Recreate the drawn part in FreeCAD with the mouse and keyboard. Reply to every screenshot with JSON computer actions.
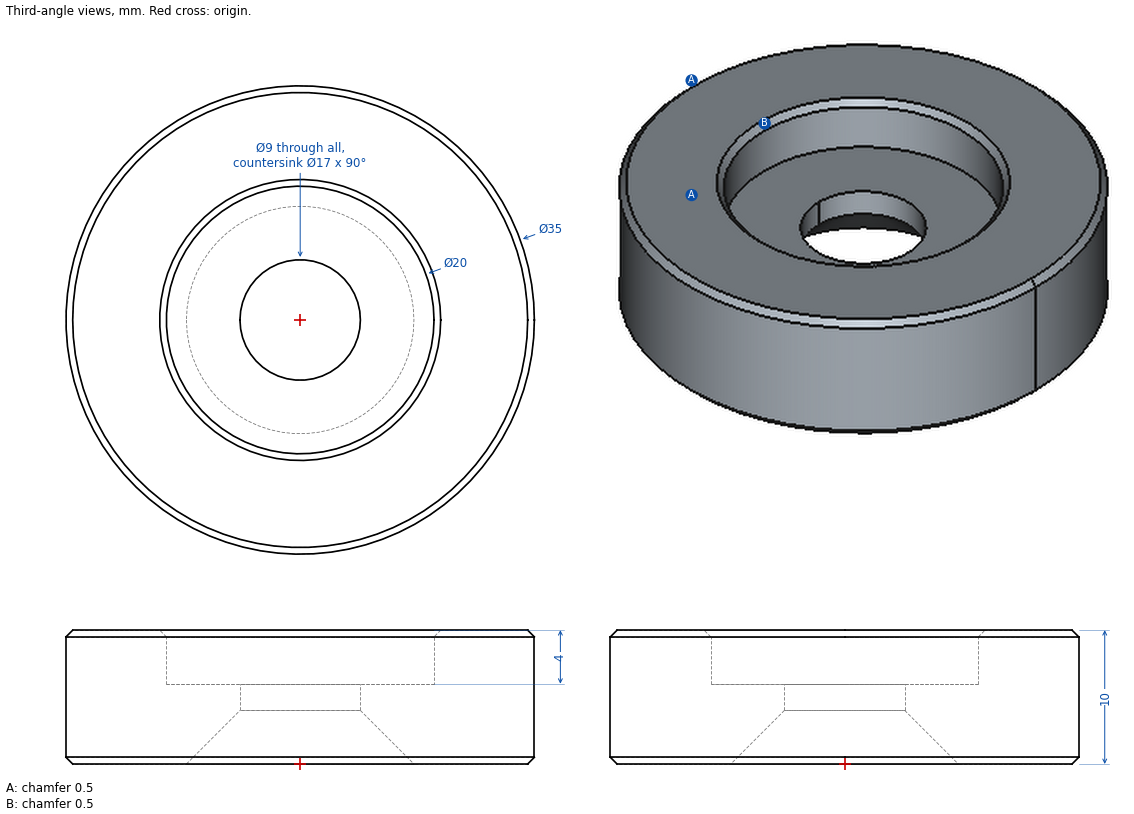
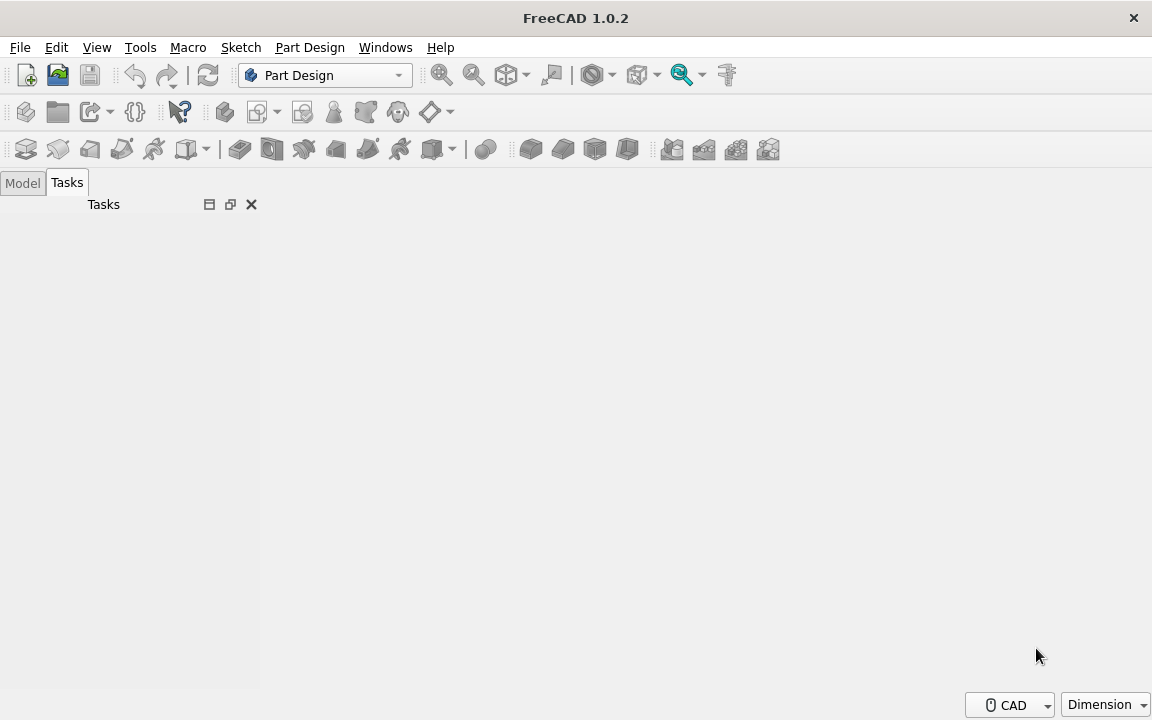
{"action": "left_click", "coordinate": [26, 76]}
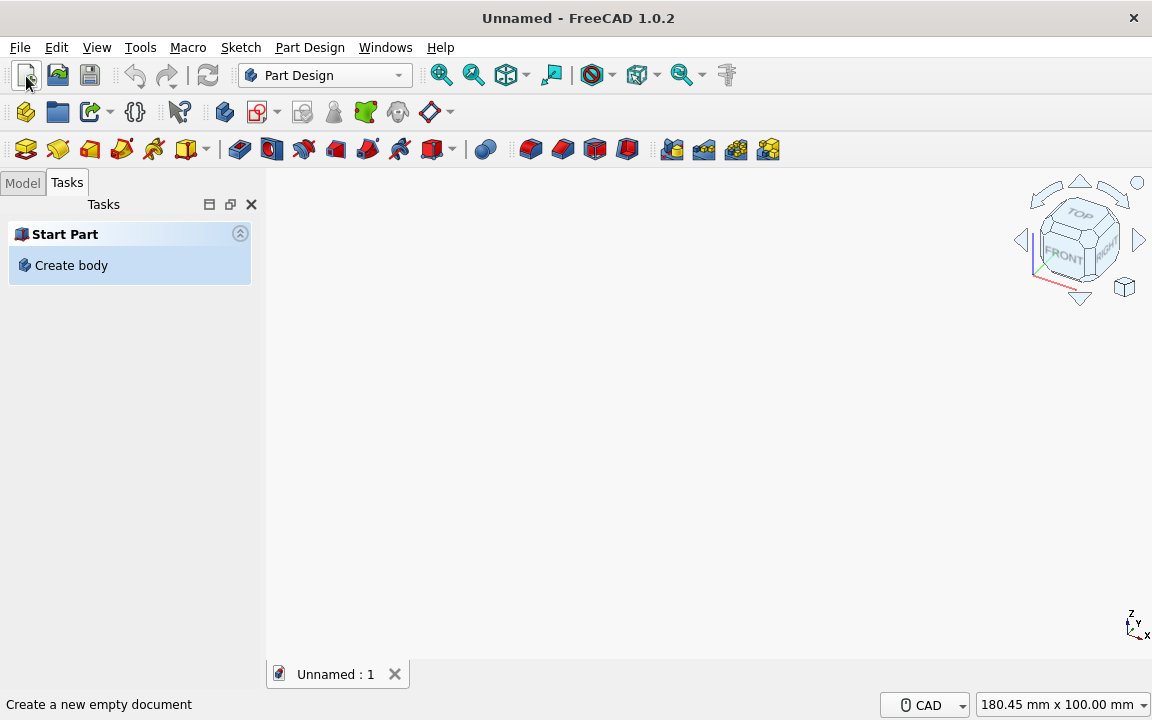
{"action": "left_click", "coordinate": [258, 112]}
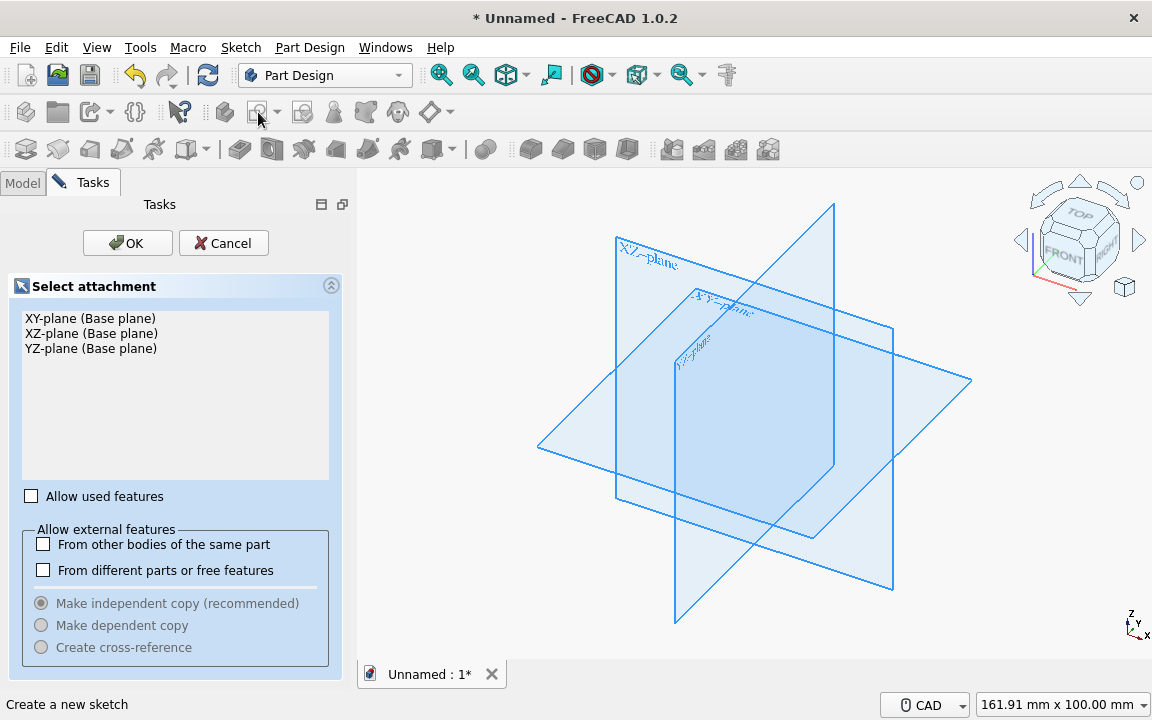
{"action": "left_click", "coordinate": [82, 318]}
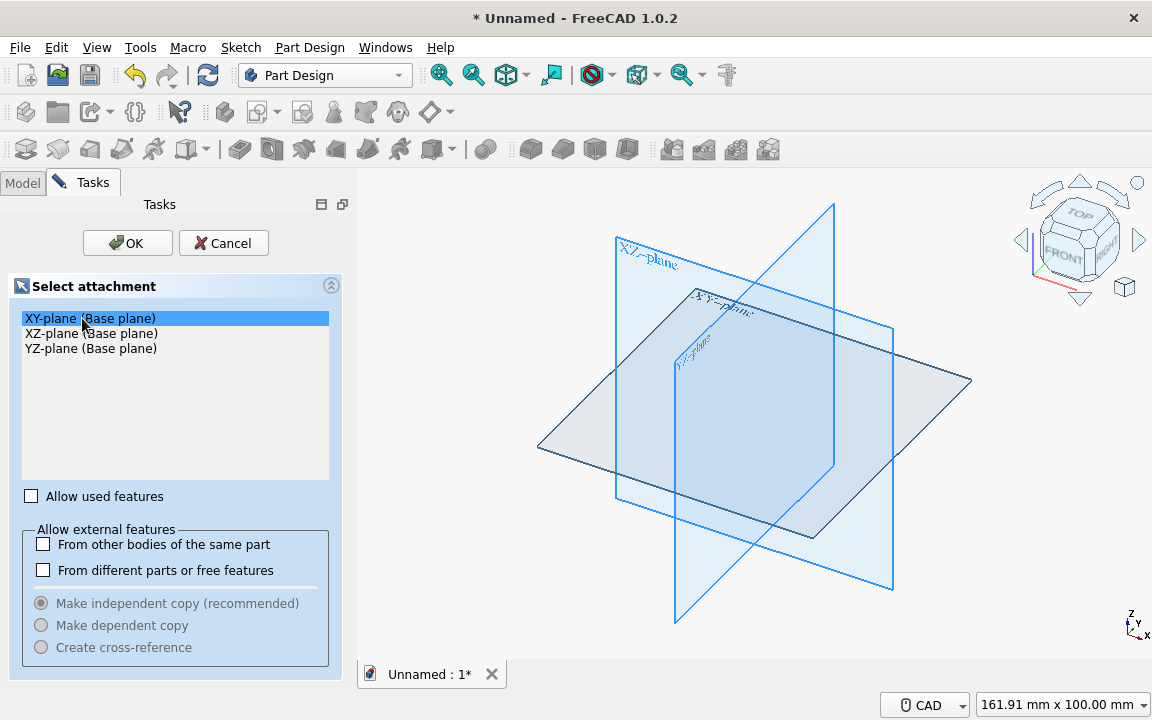
{"action": "left_click", "coordinate": [128, 243]}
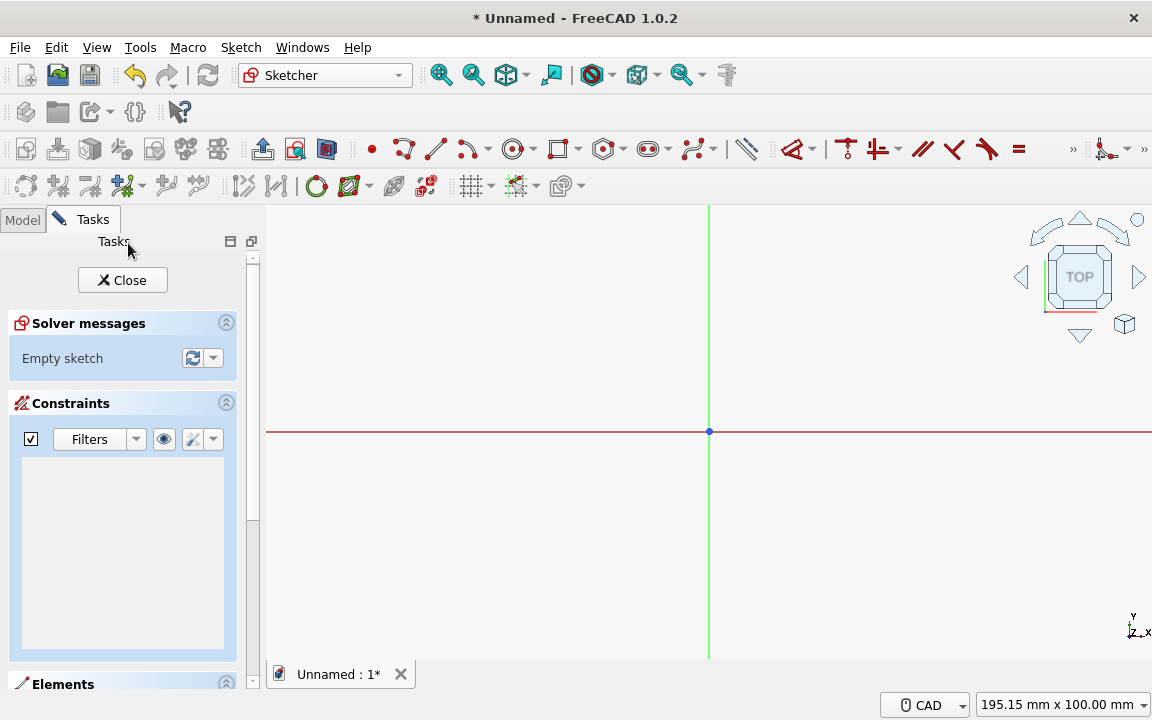
{"action": "scroll", "coordinate": [792, 432], "scroll_direction": "up", "scroll_amount": 3}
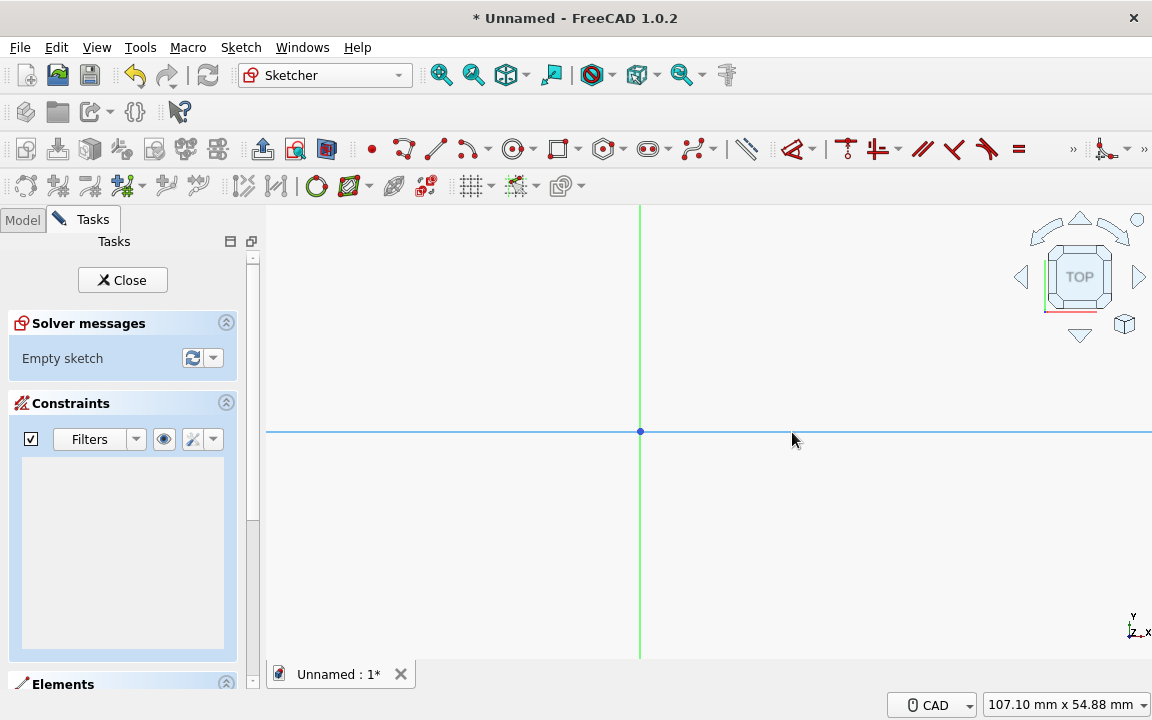
{"action": "left_click", "coordinate": [514, 150]}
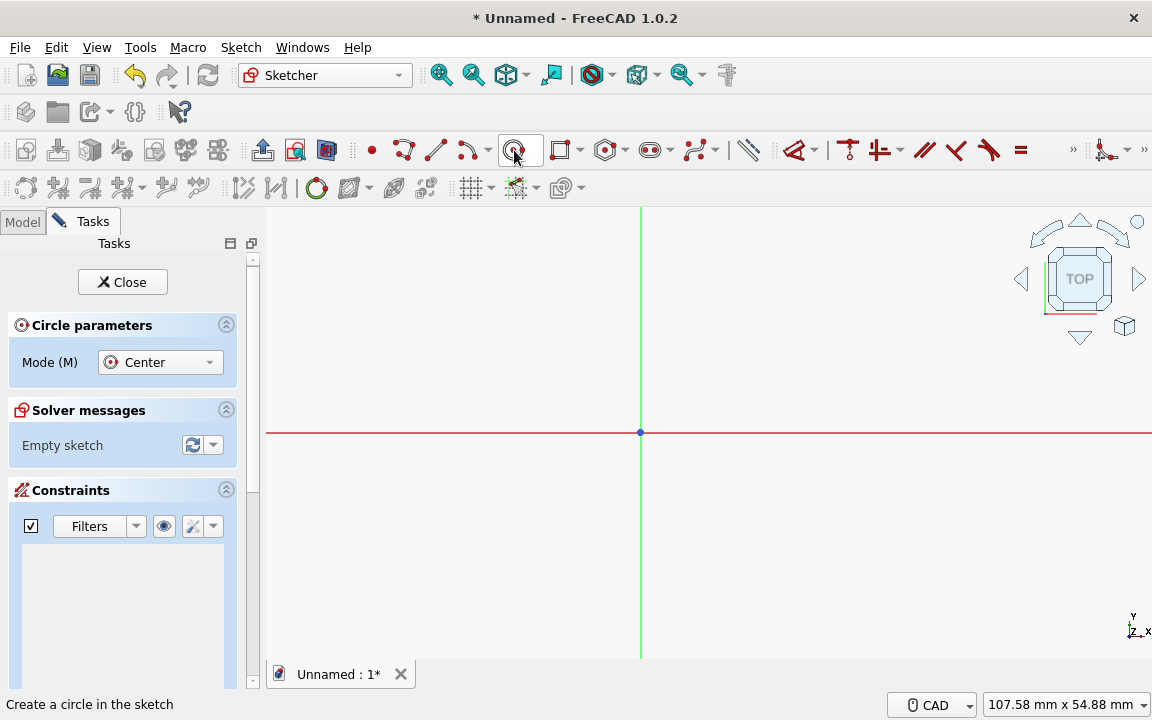
{"action": "left_click", "coordinate": [641, 433]}
{"action": "mouse_move", "coordinate": [742, 331]}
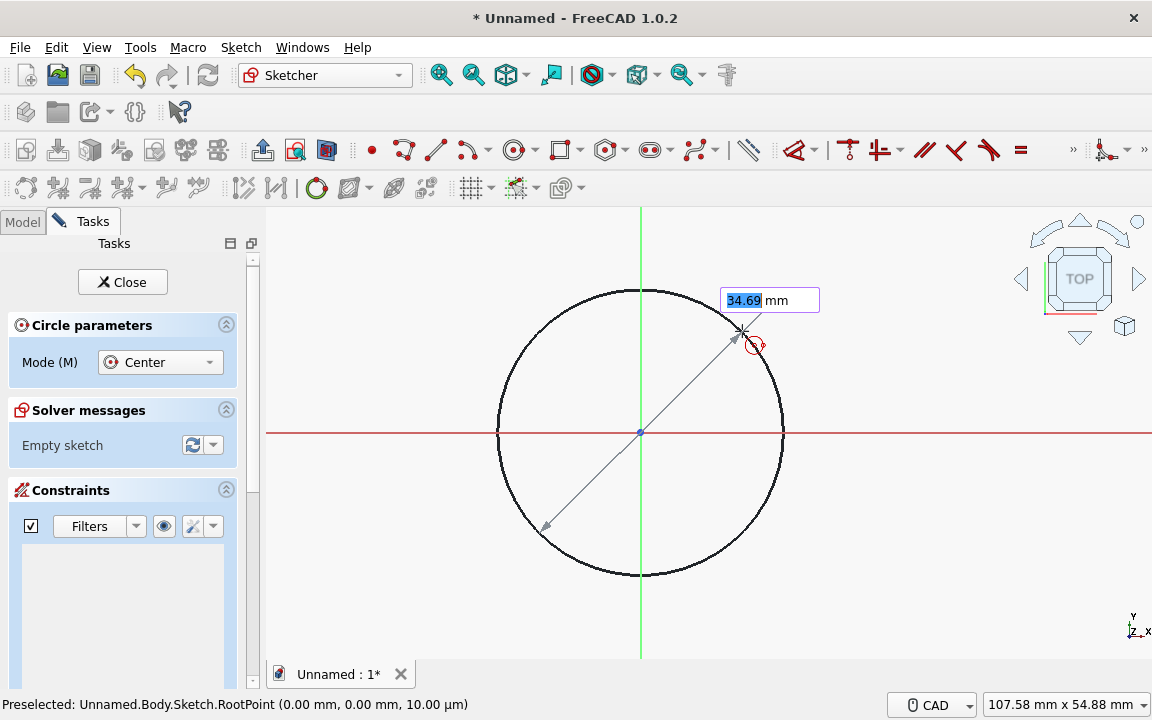
{"action": "type", "text": "35"}
{"action": "key", "text": "Return"}
{"action": "key", "text": "Escape"}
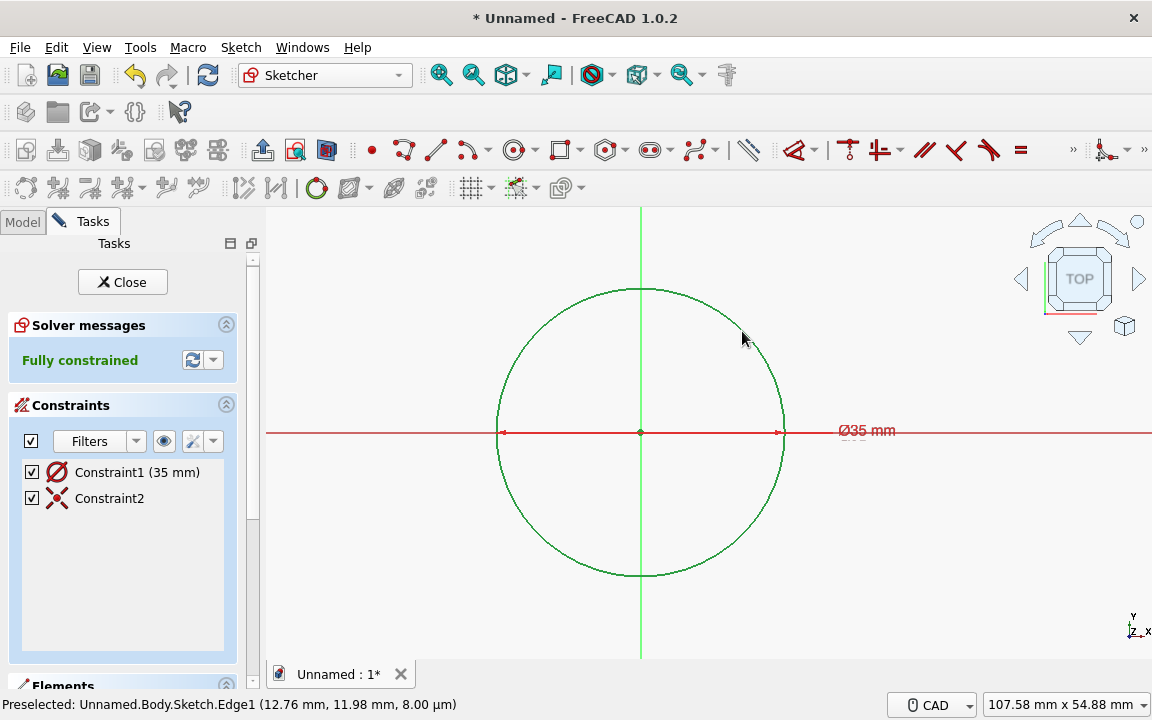
{"action": "left_click", "coordinate": [123, 282]}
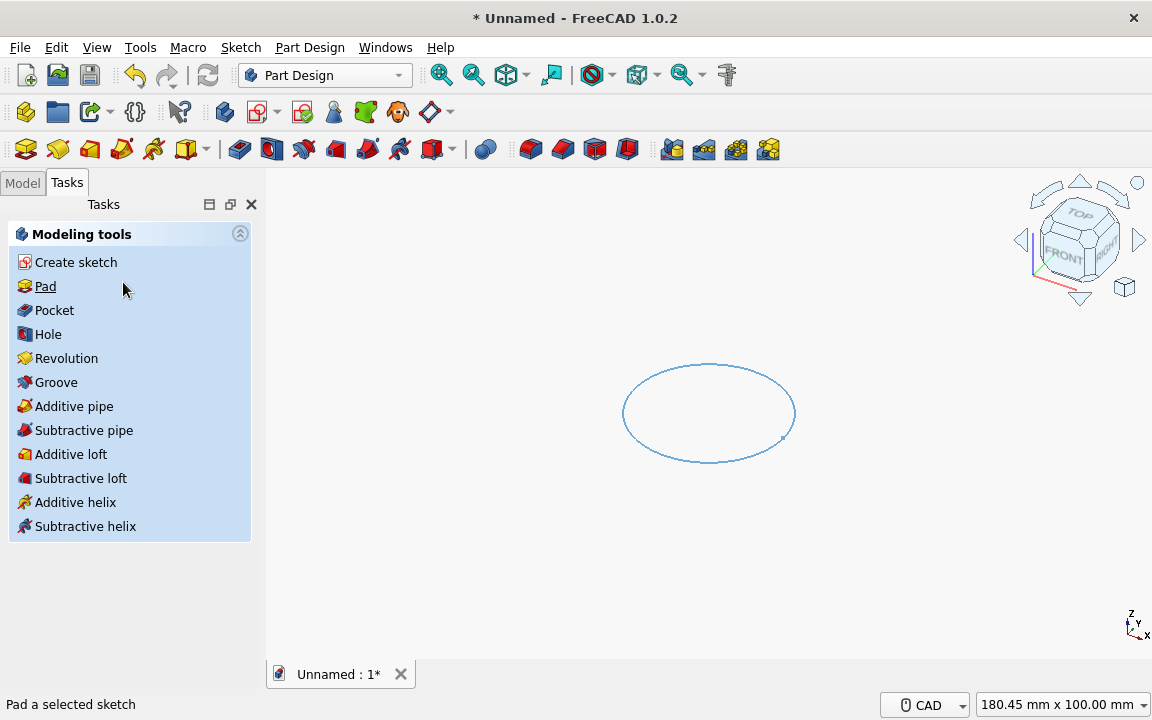
{"action": "left_click", "coordinate": [26, 150]}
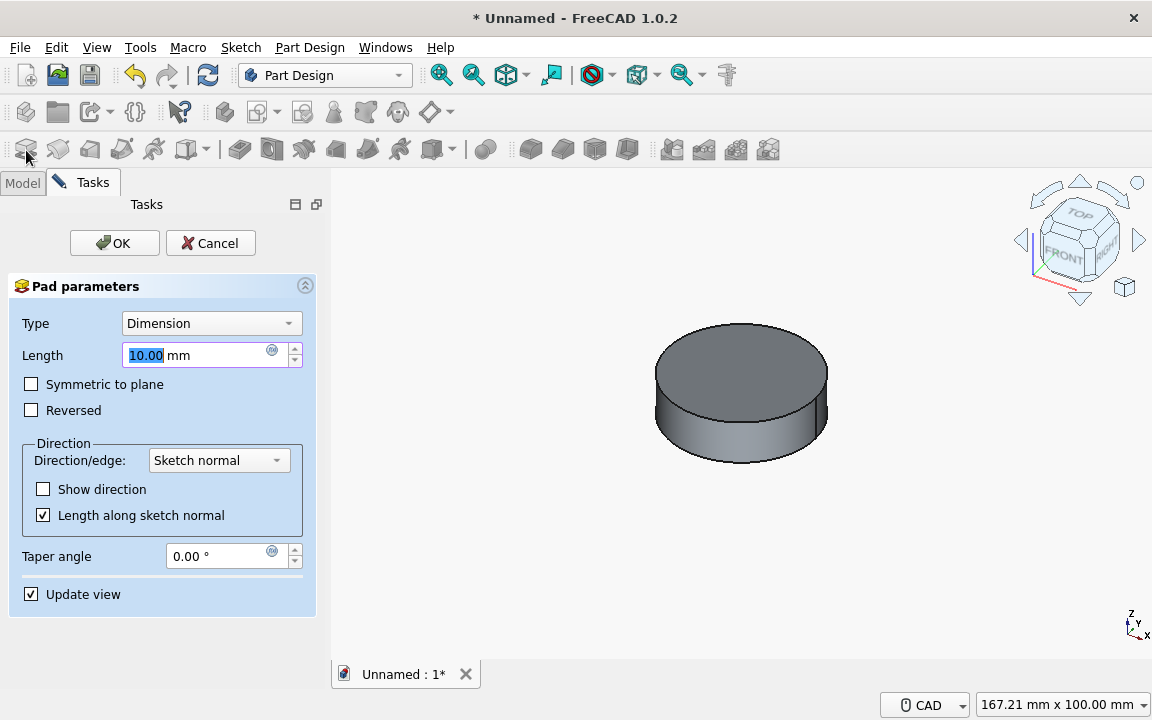
{"action": "type", "text": "10"}
{"action": "key", "text": "Tab"}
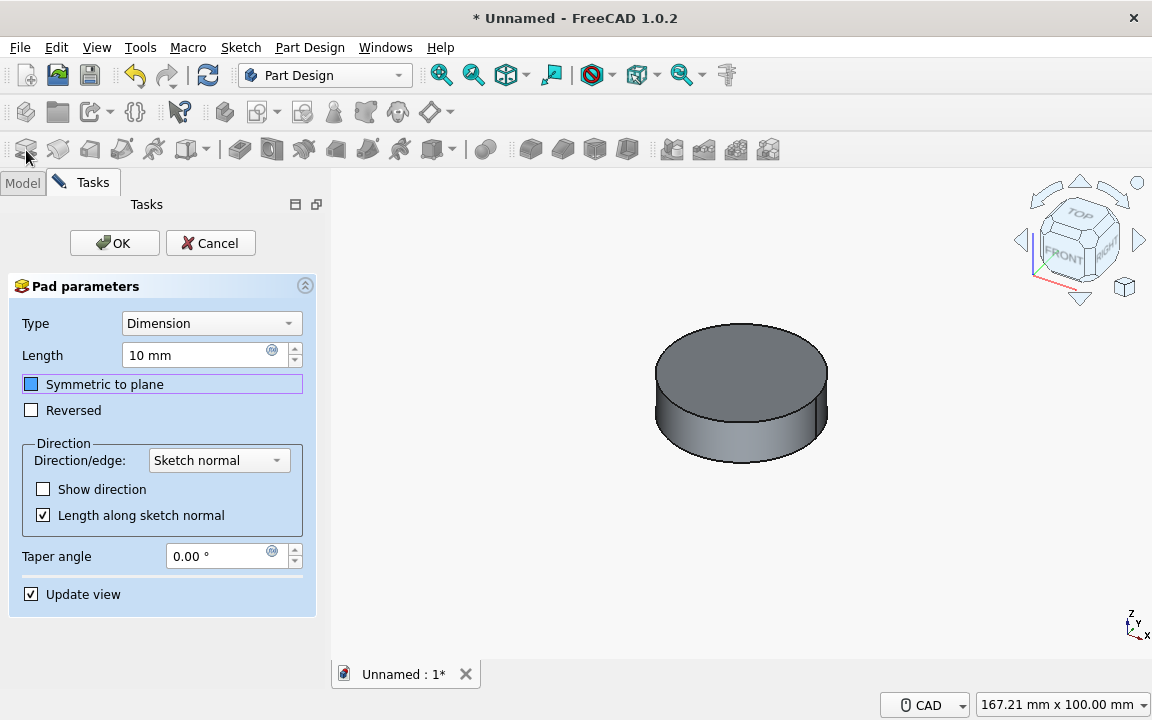
{"action": "left_click", "coordinate": [115, 243]}